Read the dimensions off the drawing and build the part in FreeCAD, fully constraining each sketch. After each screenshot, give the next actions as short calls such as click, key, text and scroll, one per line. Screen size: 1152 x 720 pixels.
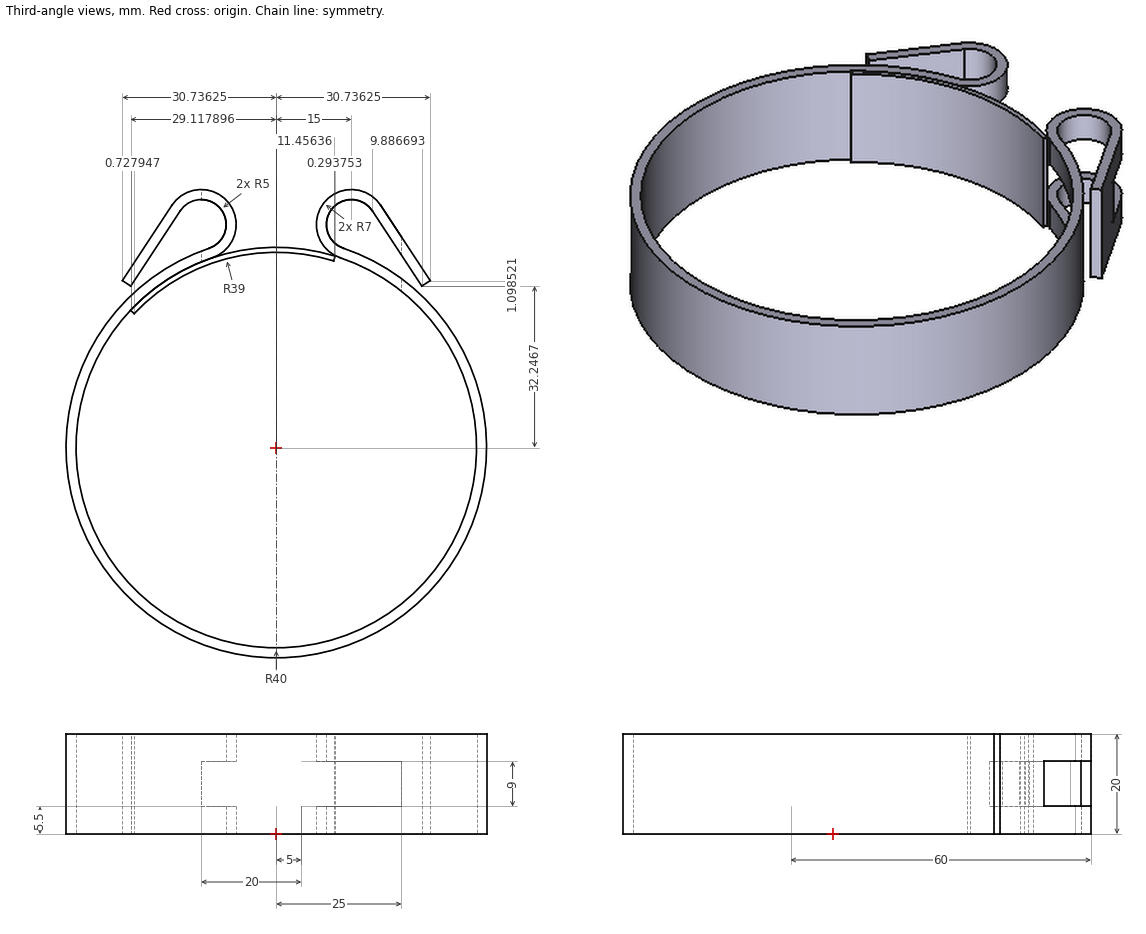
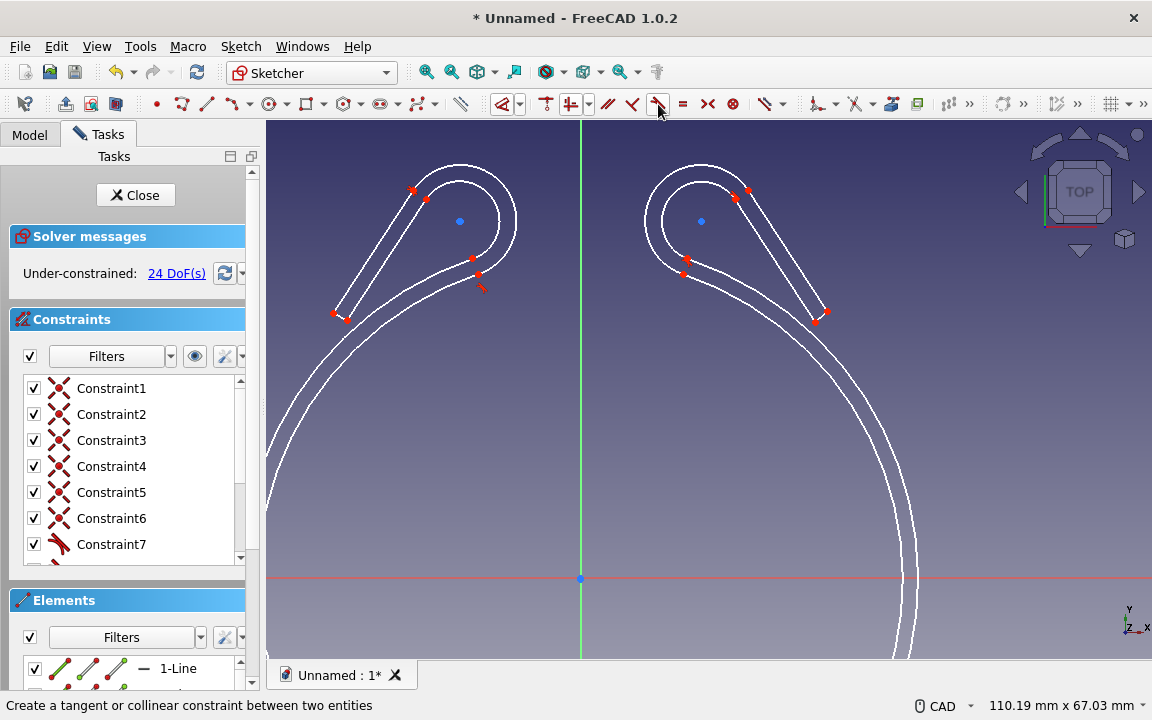
click(499, 225)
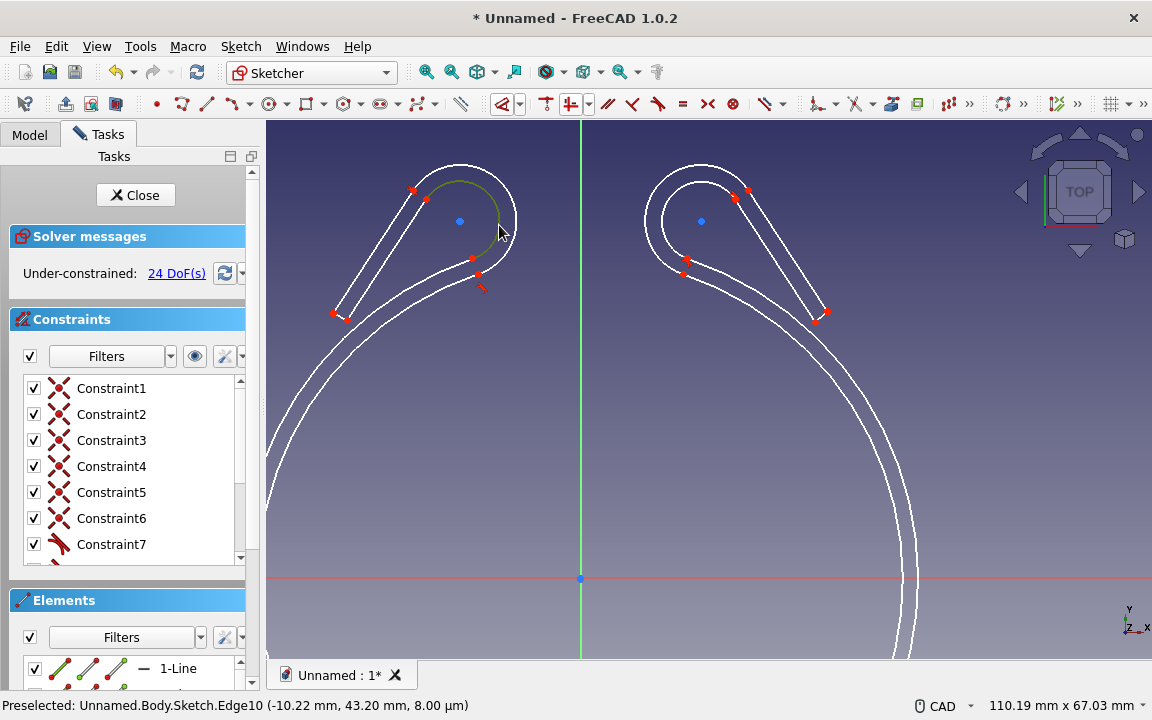
click(916, 539)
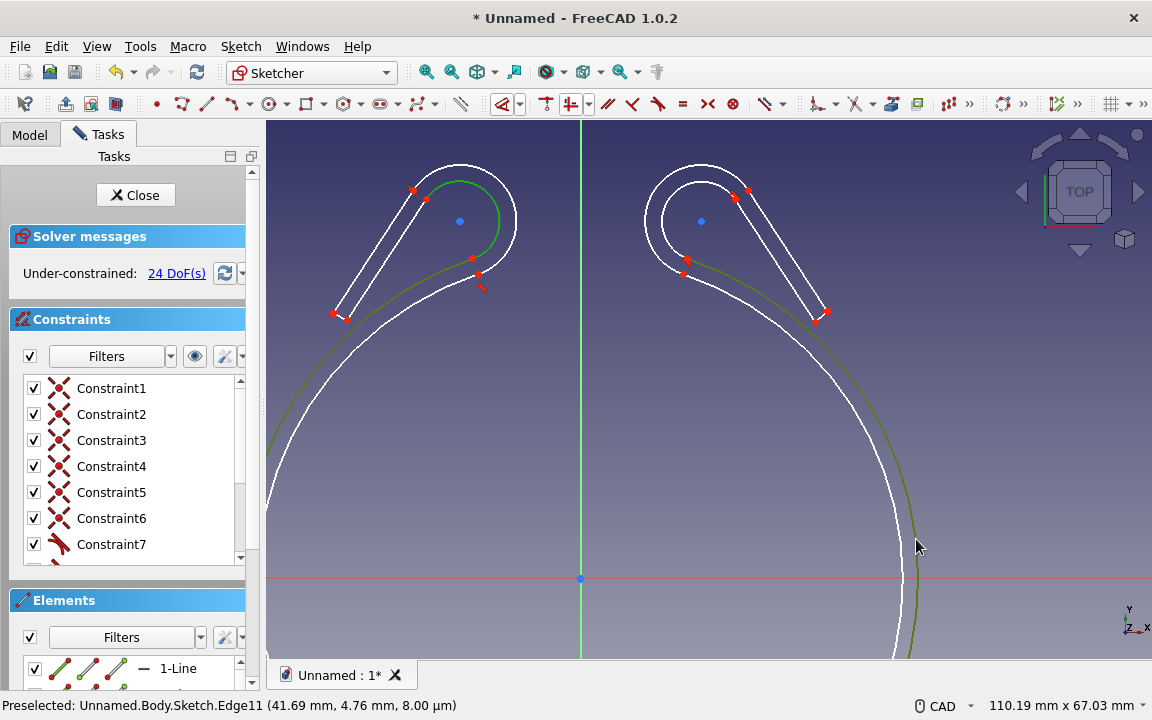
key(t)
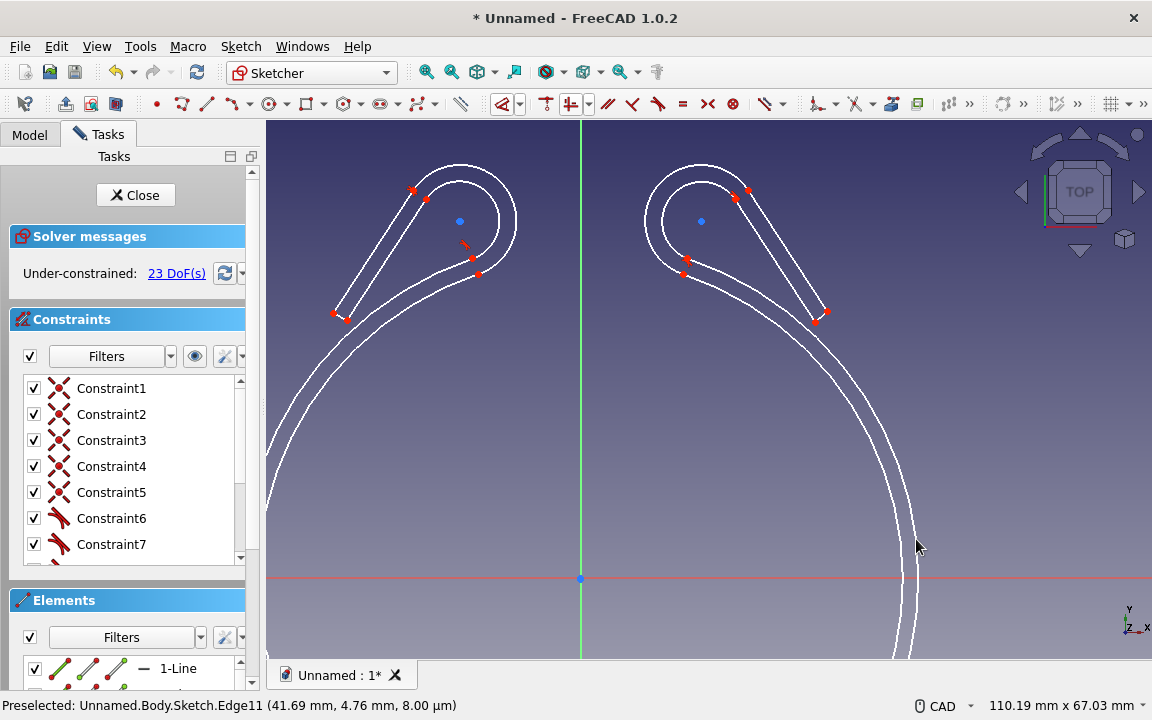
click(916, 539)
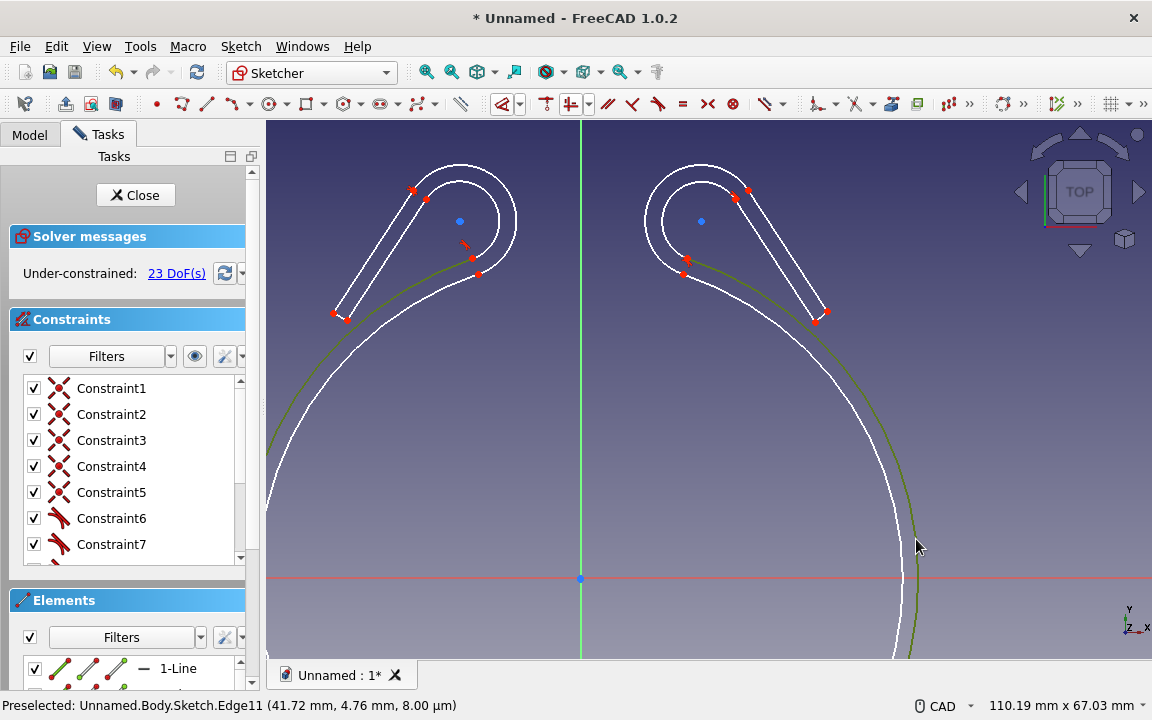
click(696, 182)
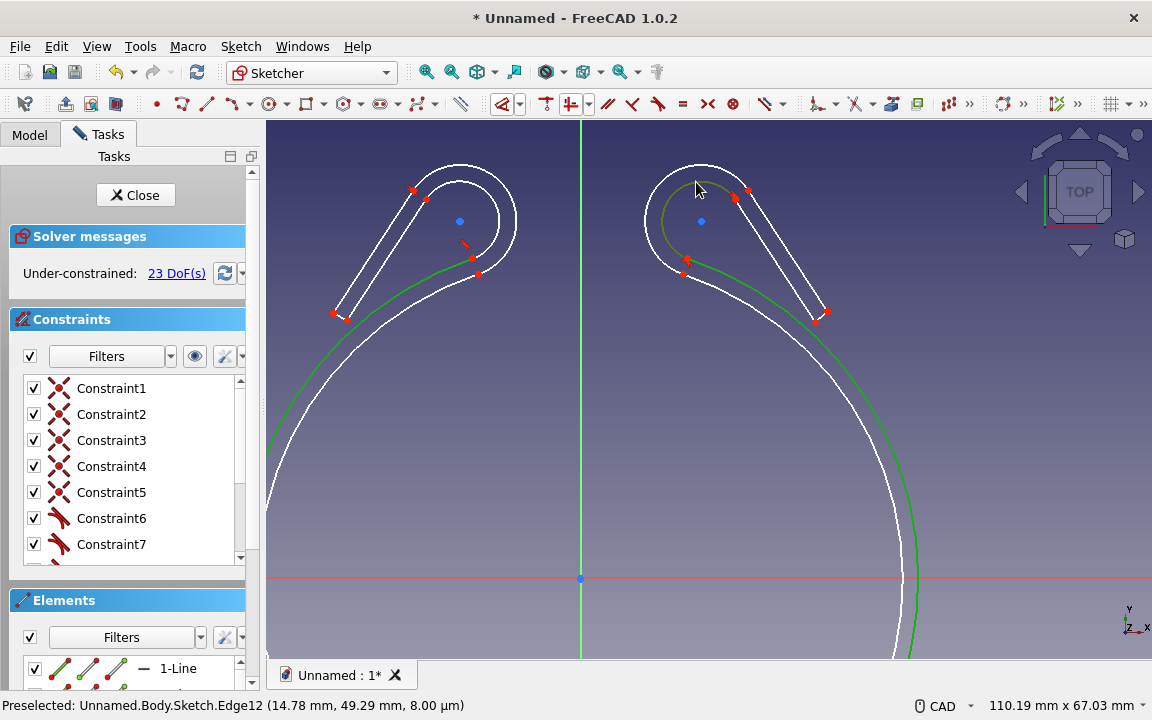
key(t)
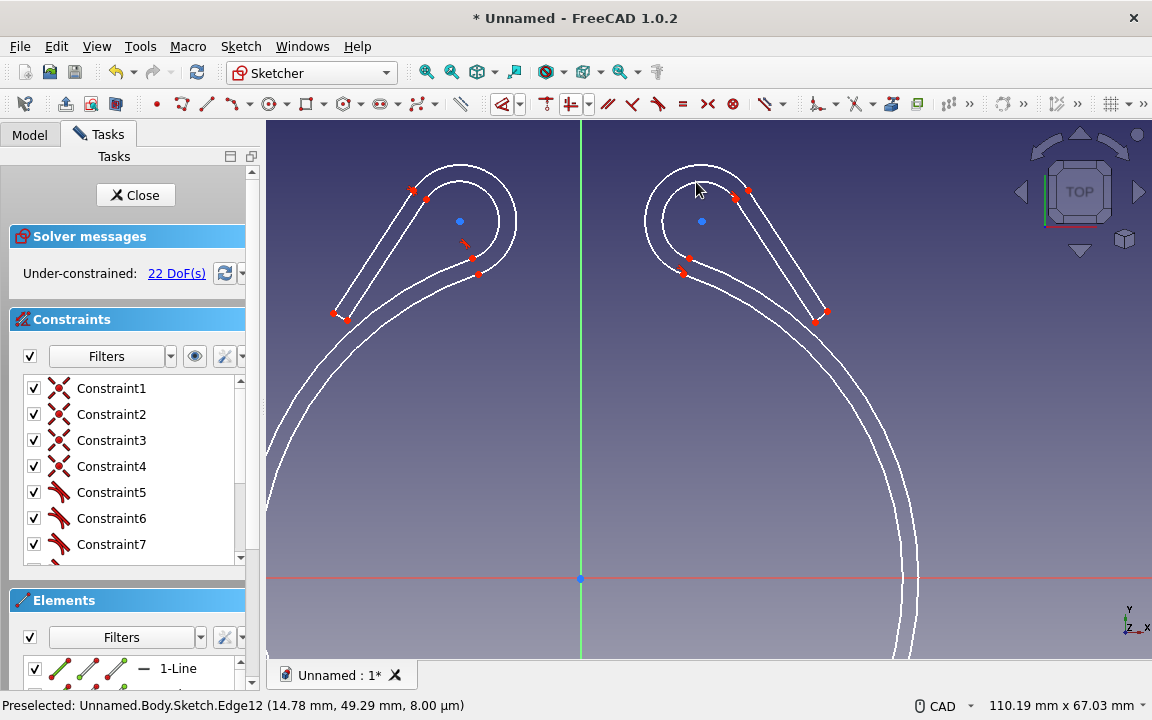
click(516, 227)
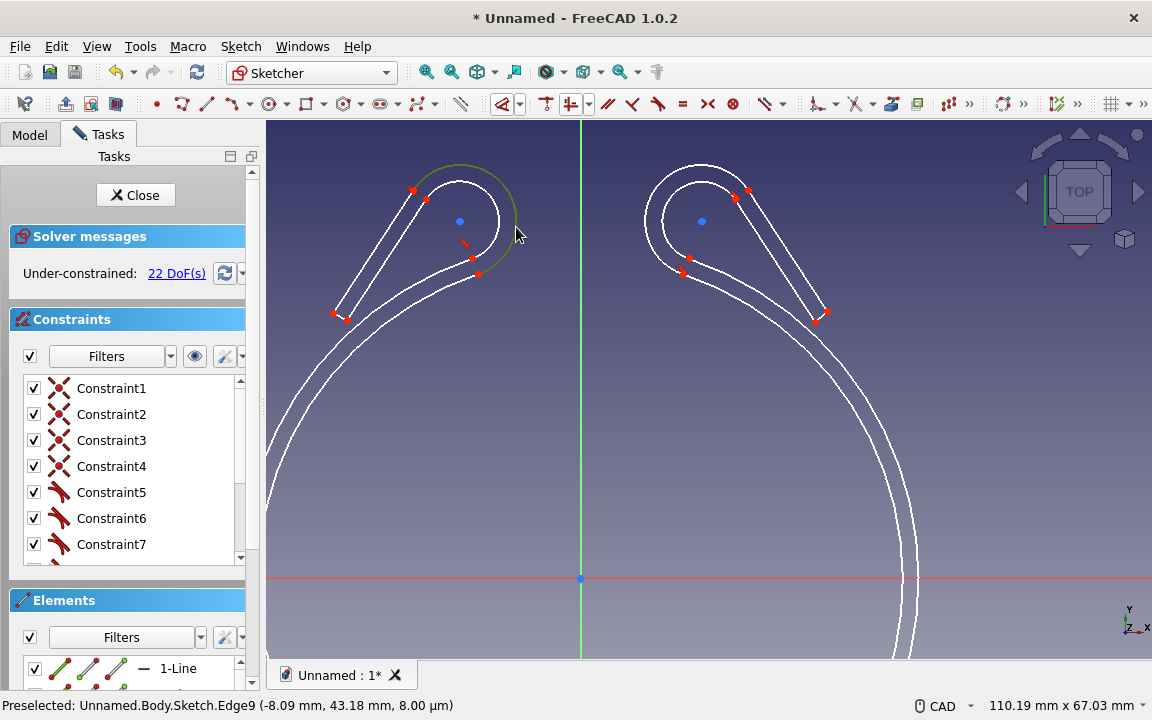
click(499, 225)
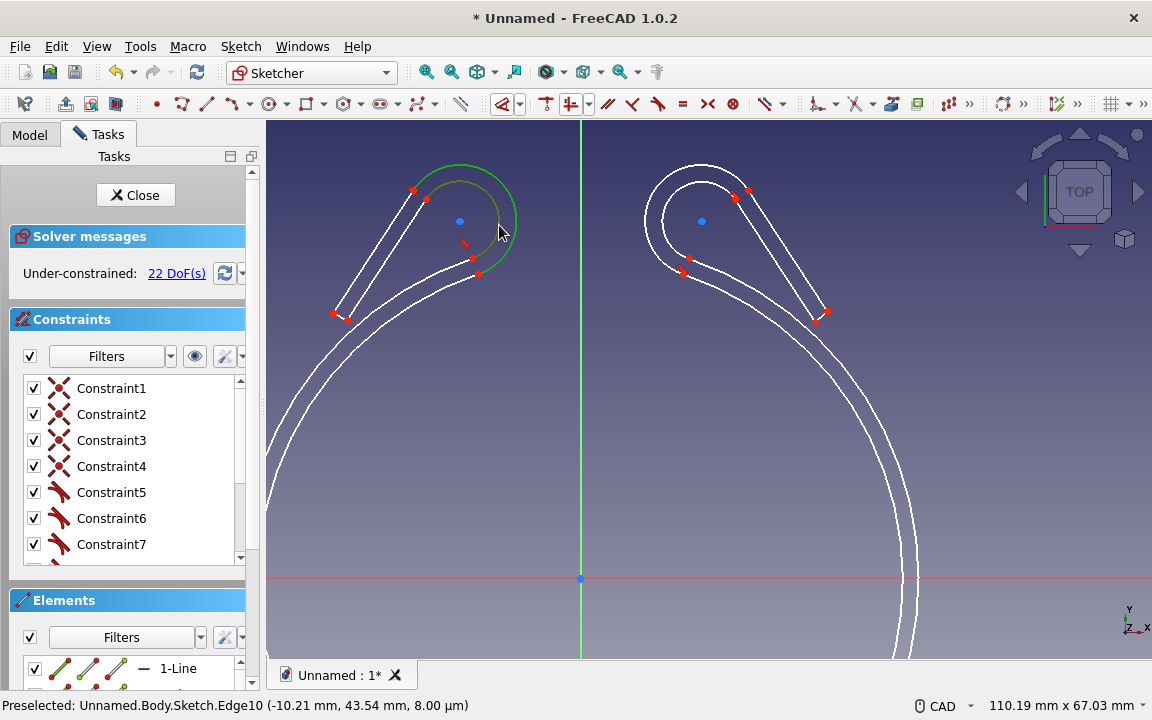
key(c)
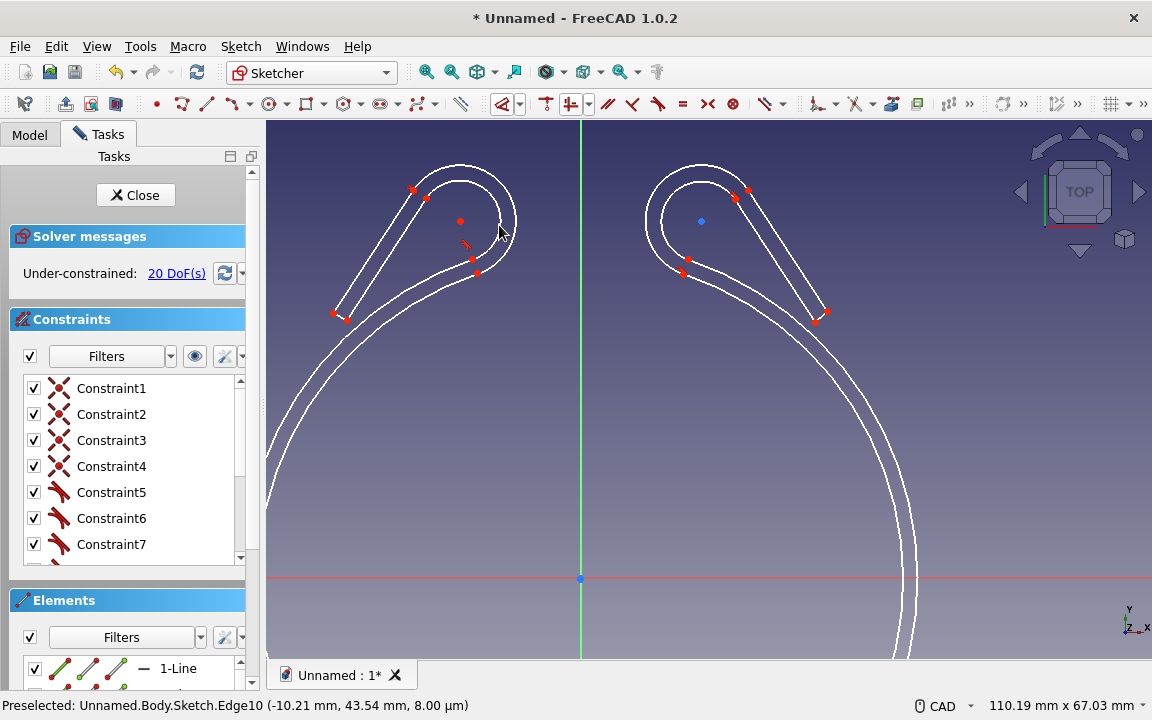
click(901, 542)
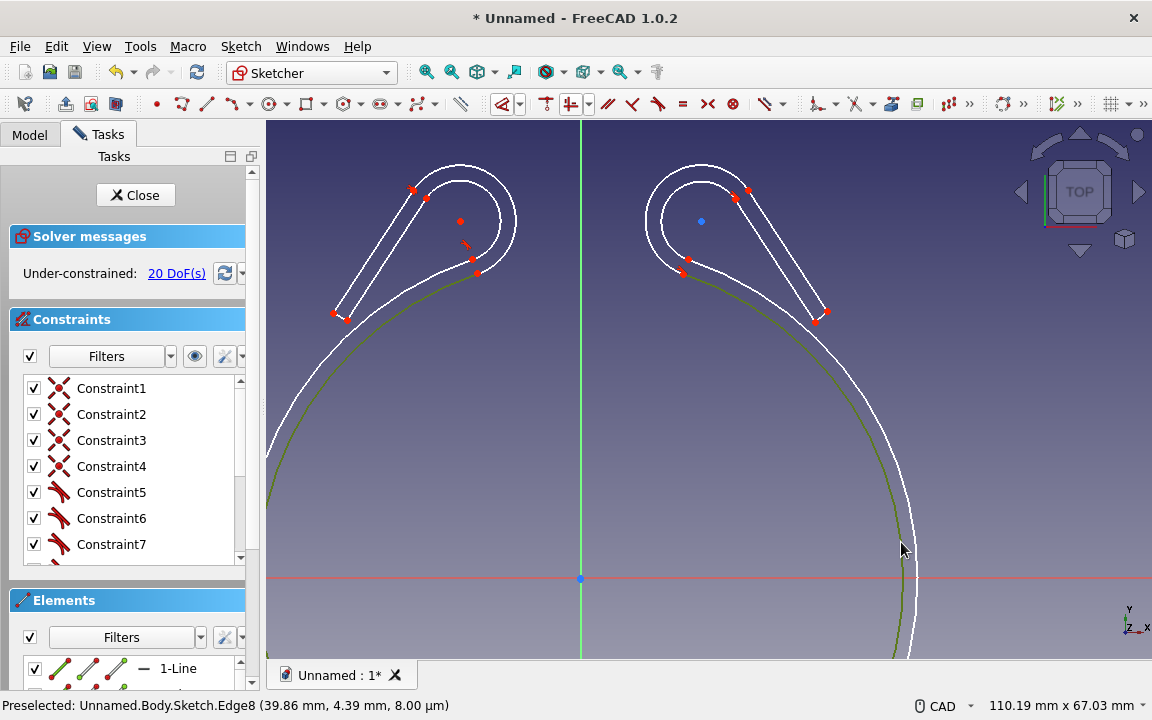
click(915, 540)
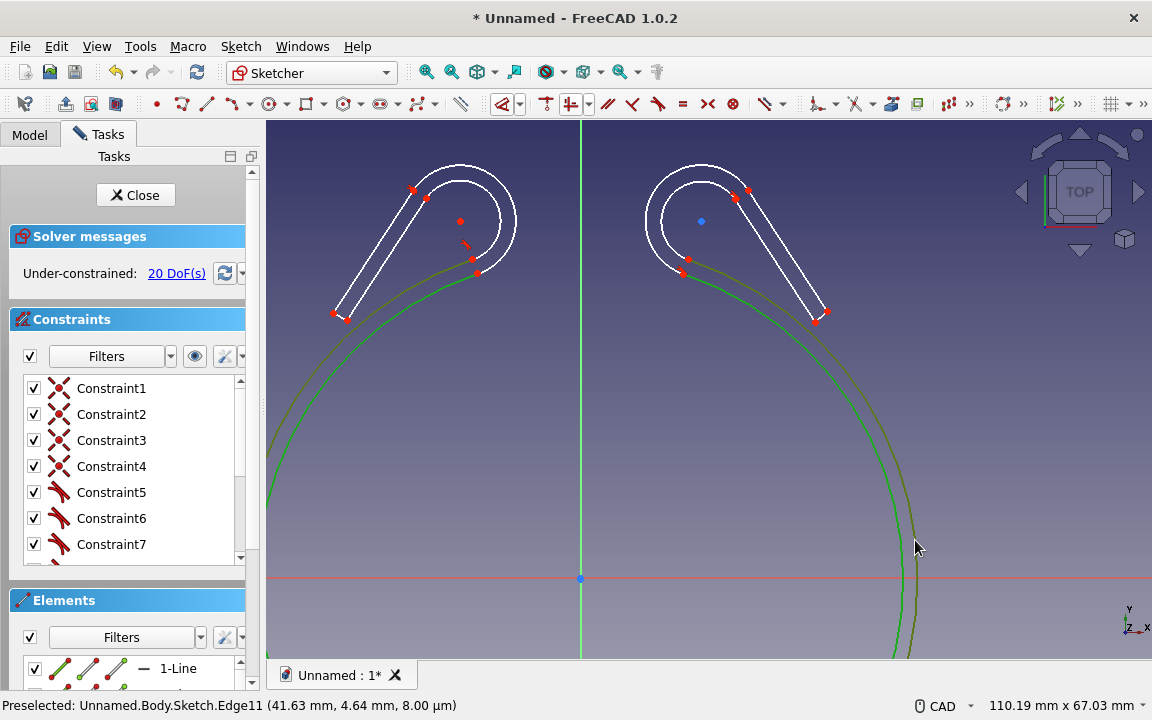
key(c)